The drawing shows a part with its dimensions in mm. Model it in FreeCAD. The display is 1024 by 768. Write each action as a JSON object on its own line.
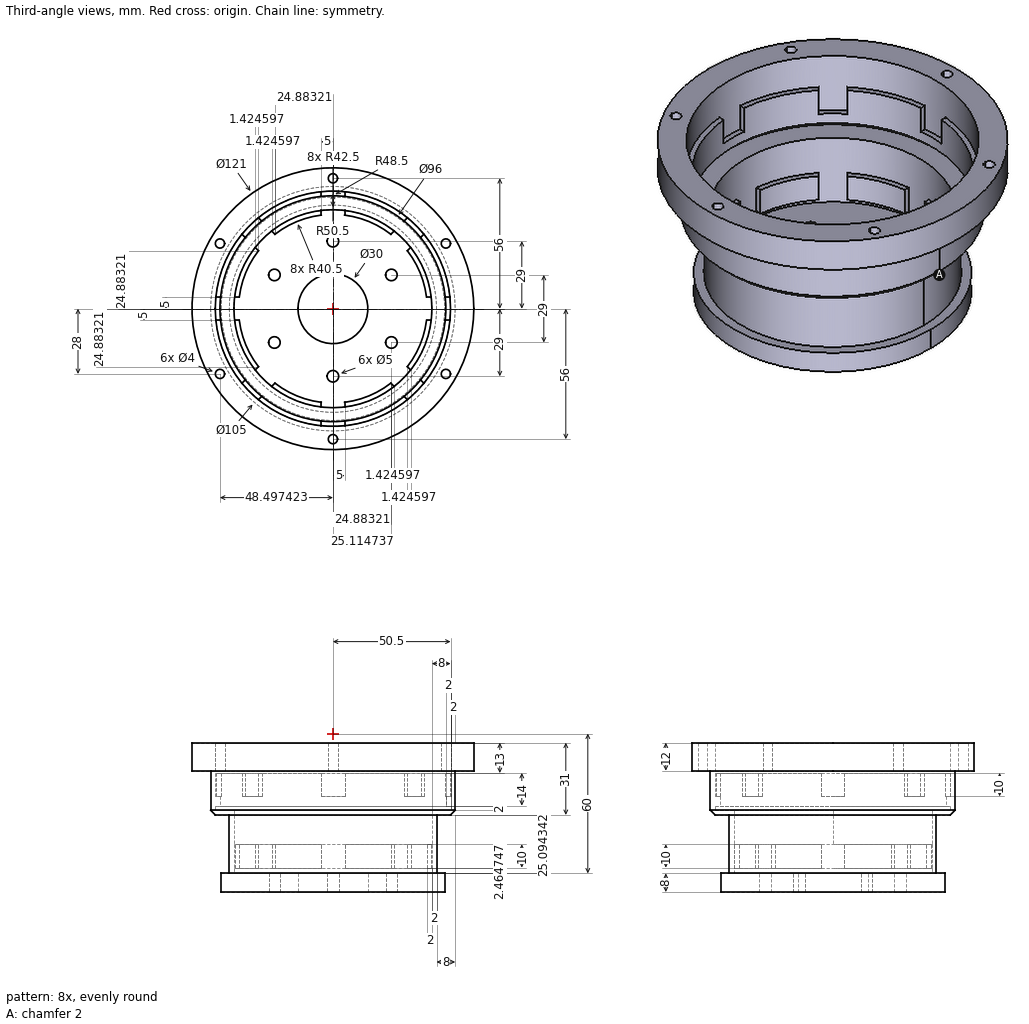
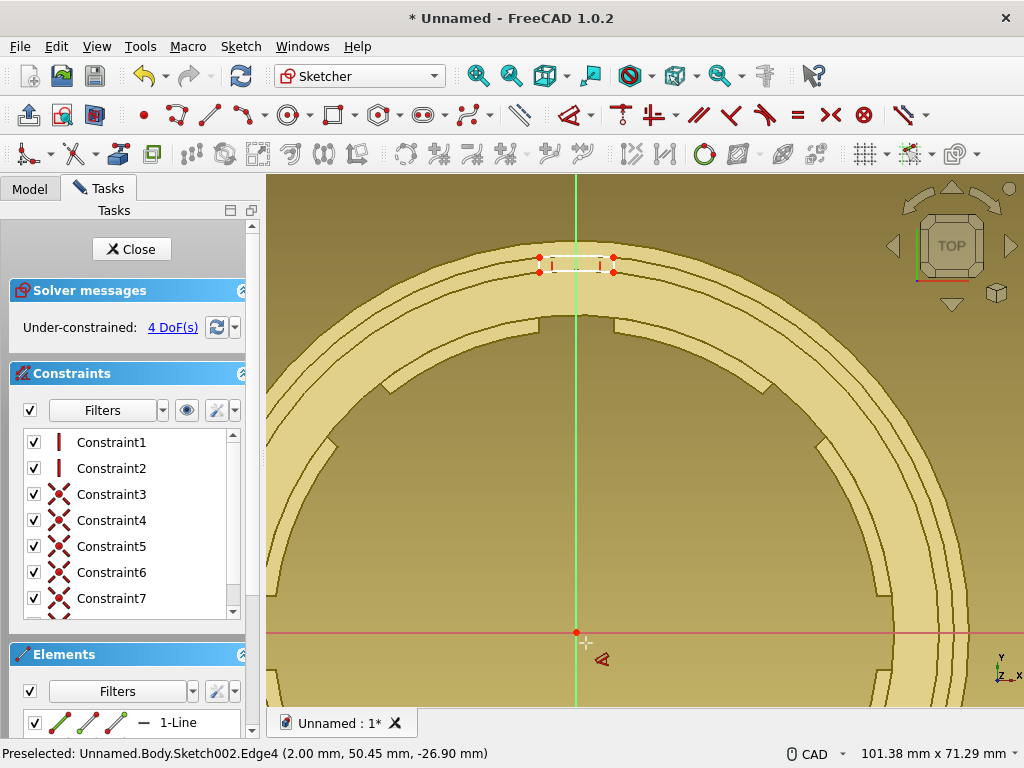
{"action": "left_click", "coordinate": [591, 271]}
{"action": "left_click", "coordinate": [592, 239]}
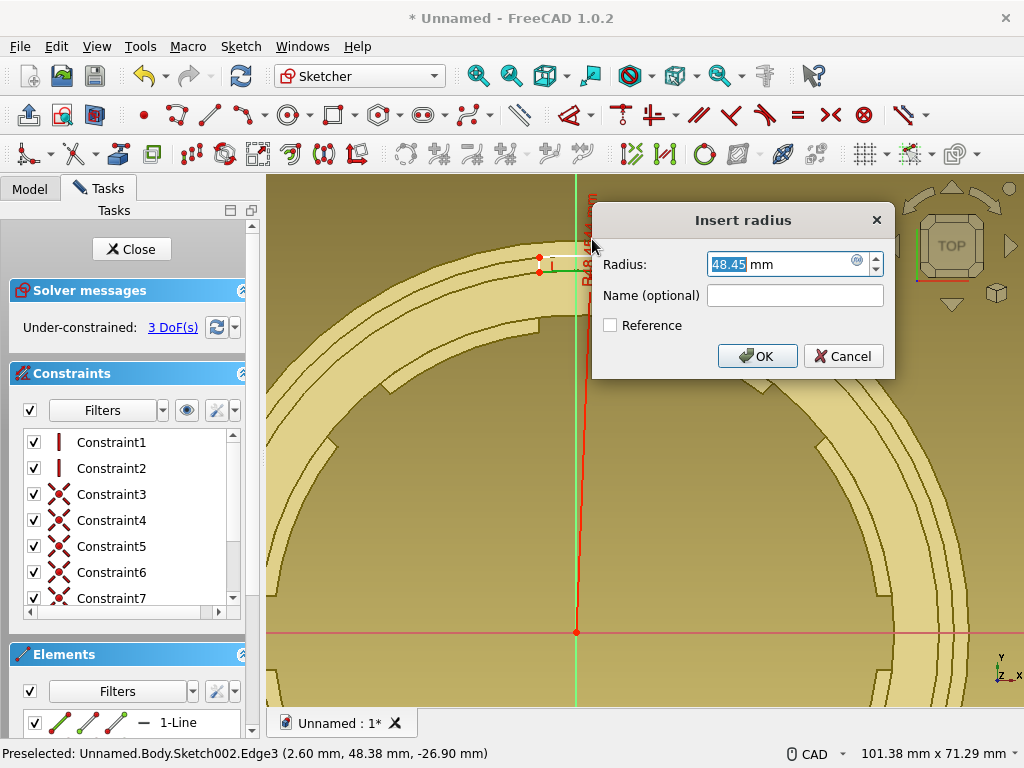
{"action": "type", "text": "48.5"}
{"action": "key", "text": "Return"}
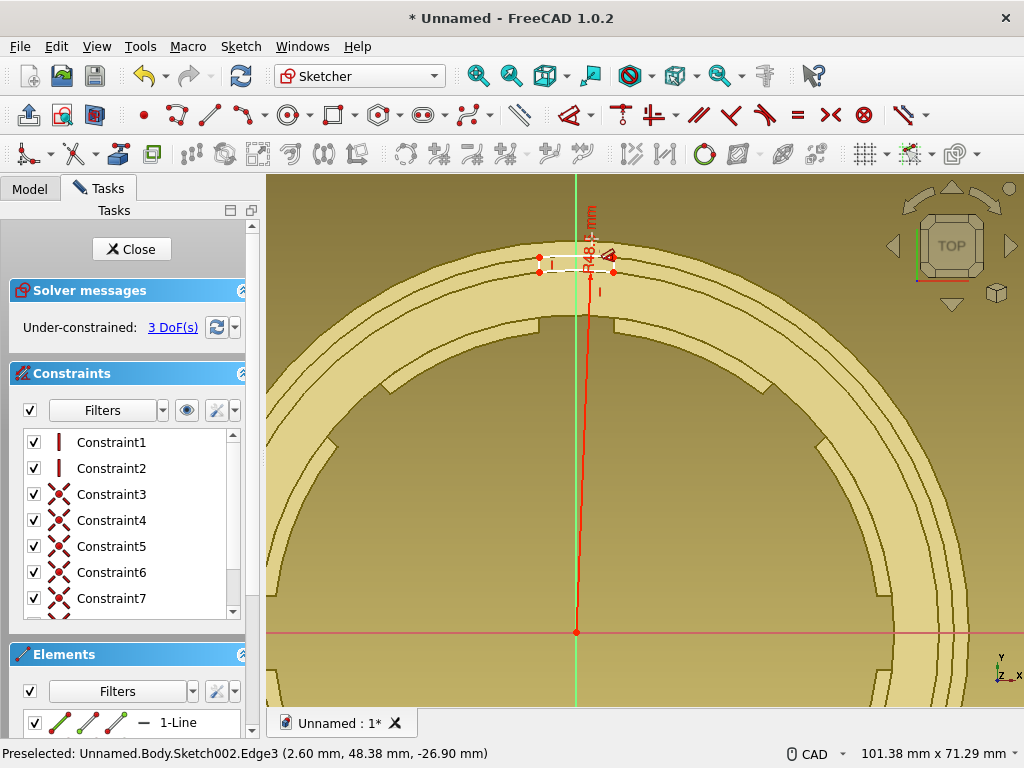
{"action": "left_click", "coordinate": [591, 256]}
{"action": "left_click", "coordinate": [786, 282]}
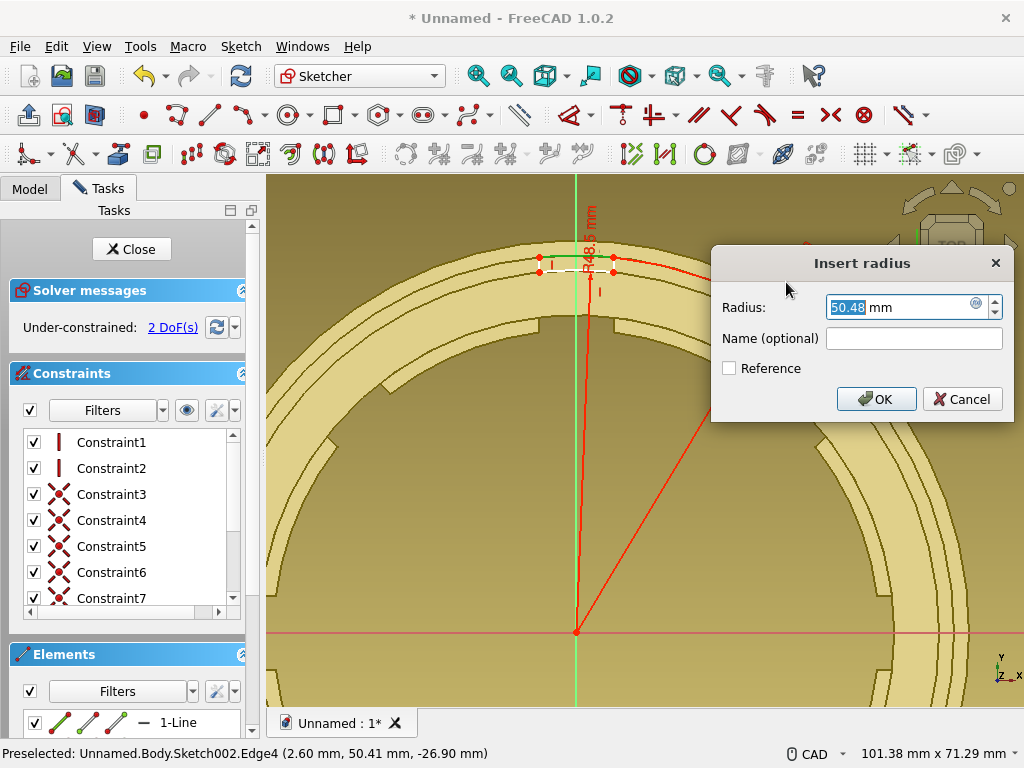
{"action": "type", "text": "50.5"}
{"action": "key", "text": "Return"}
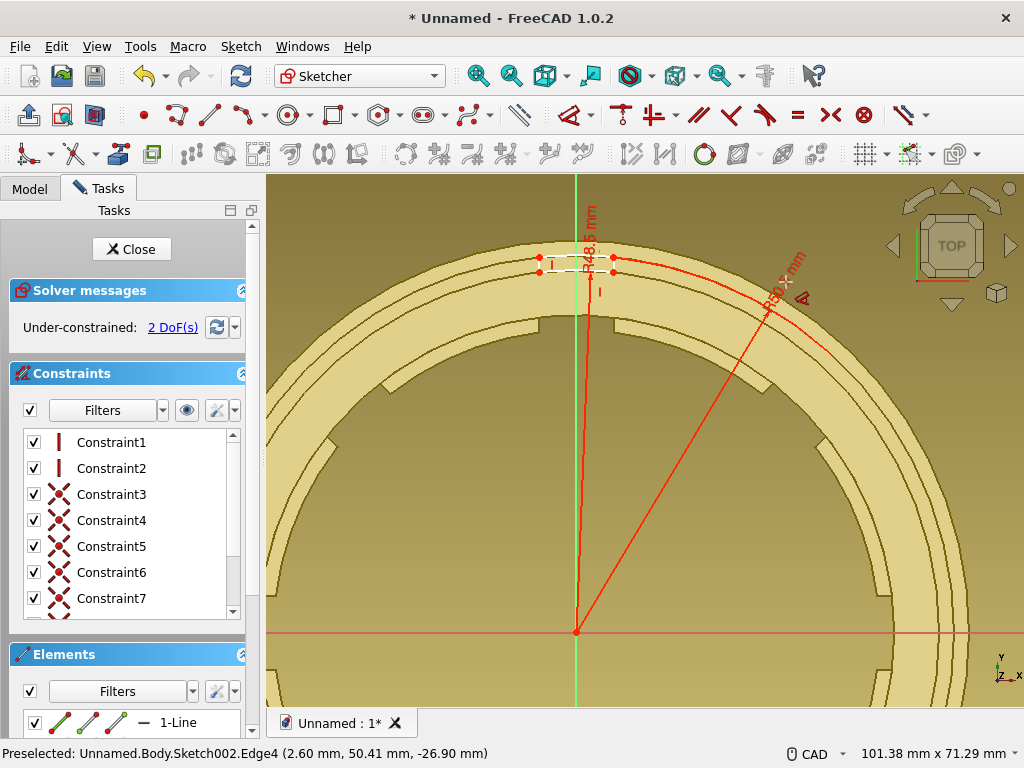
{"action": "left_click", "coordinate": [539, 257]}
{"action": "left_click", "coordinate": [558, 667]}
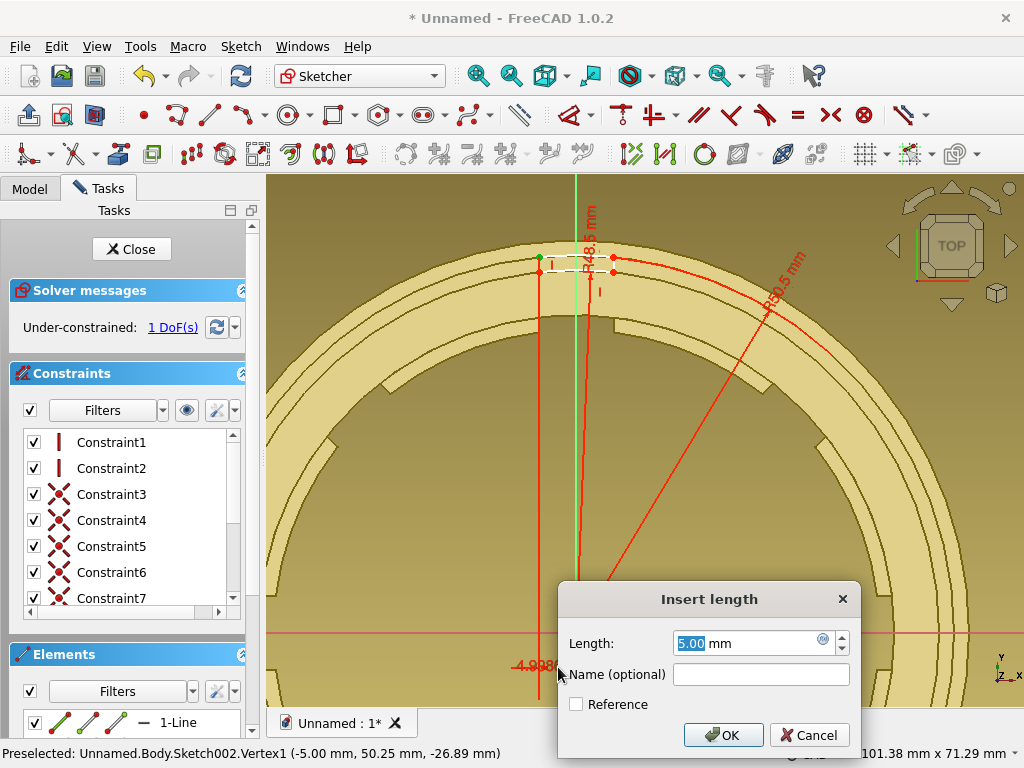
{"action": "type", "text": "5"}
{"action": "key", "text": "Return"}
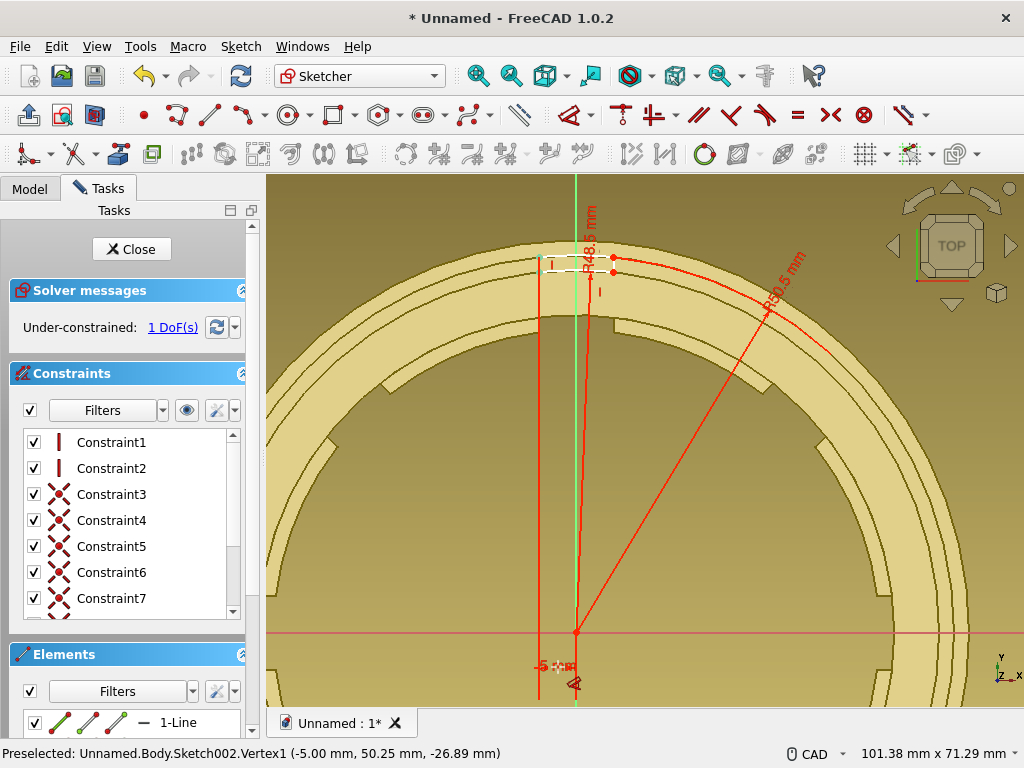
{"action": "left_click", "coordinate": [614, 272]}
{"action": "left_click", "coordinate": [595, 214]}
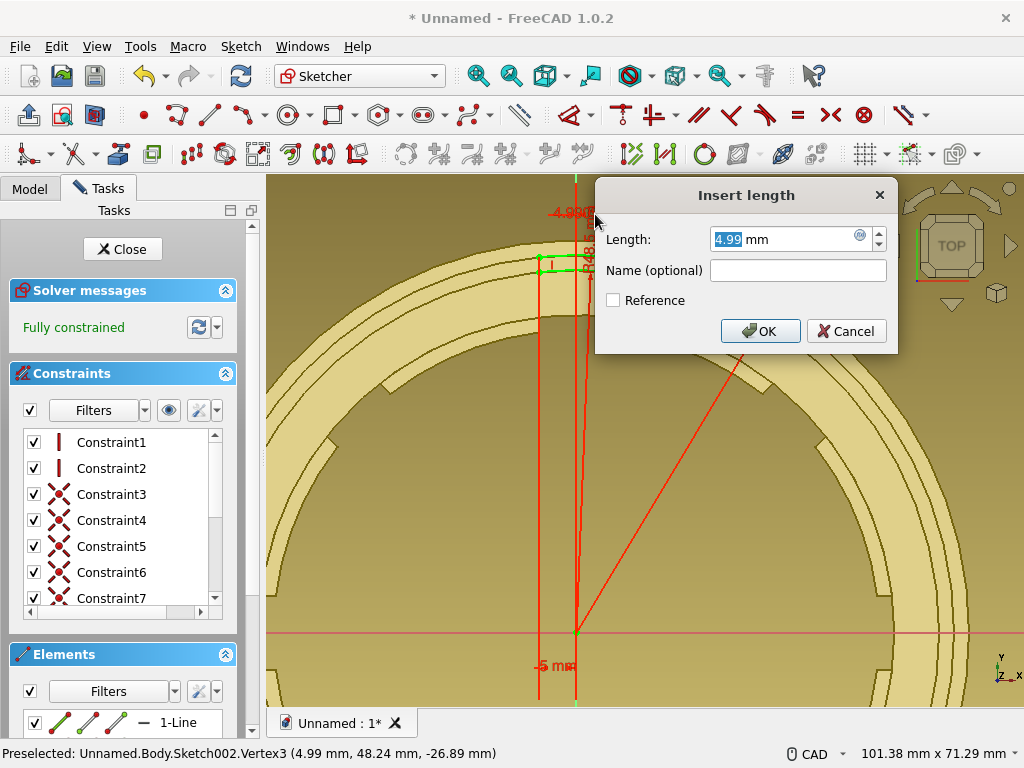
{"action": "type", "text": "5"}
{"action": "key", "text": "Return"}
{"action": "key", "text": "Escape"}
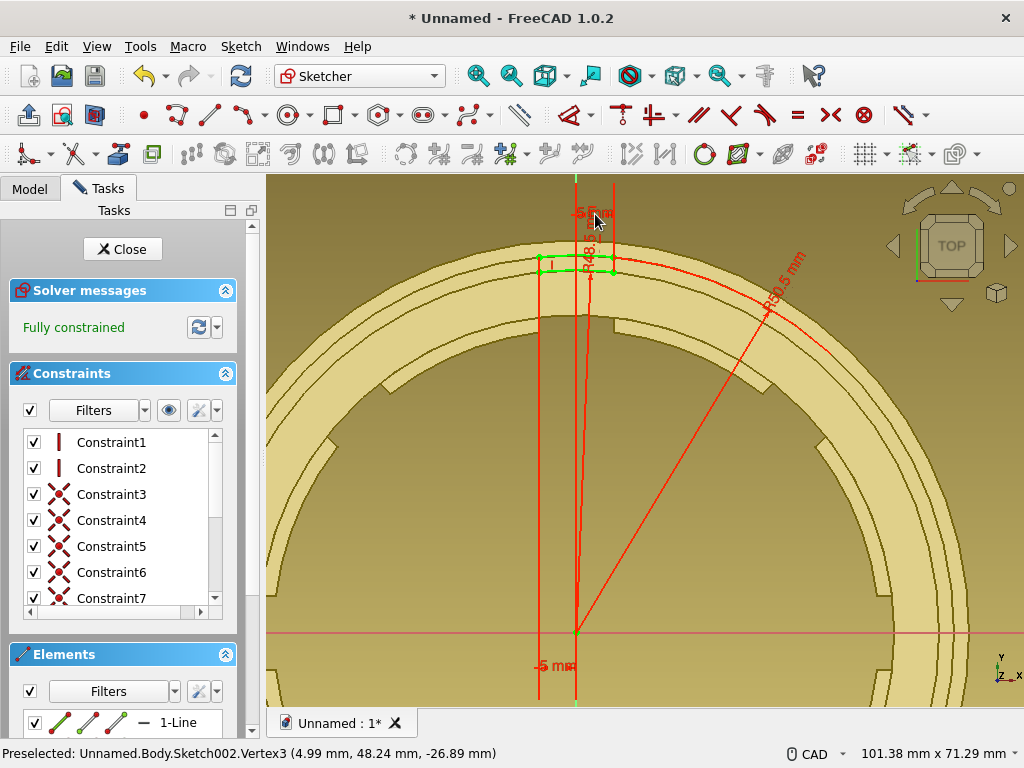
{"action": "left_click", "coordinate": [123, 249]}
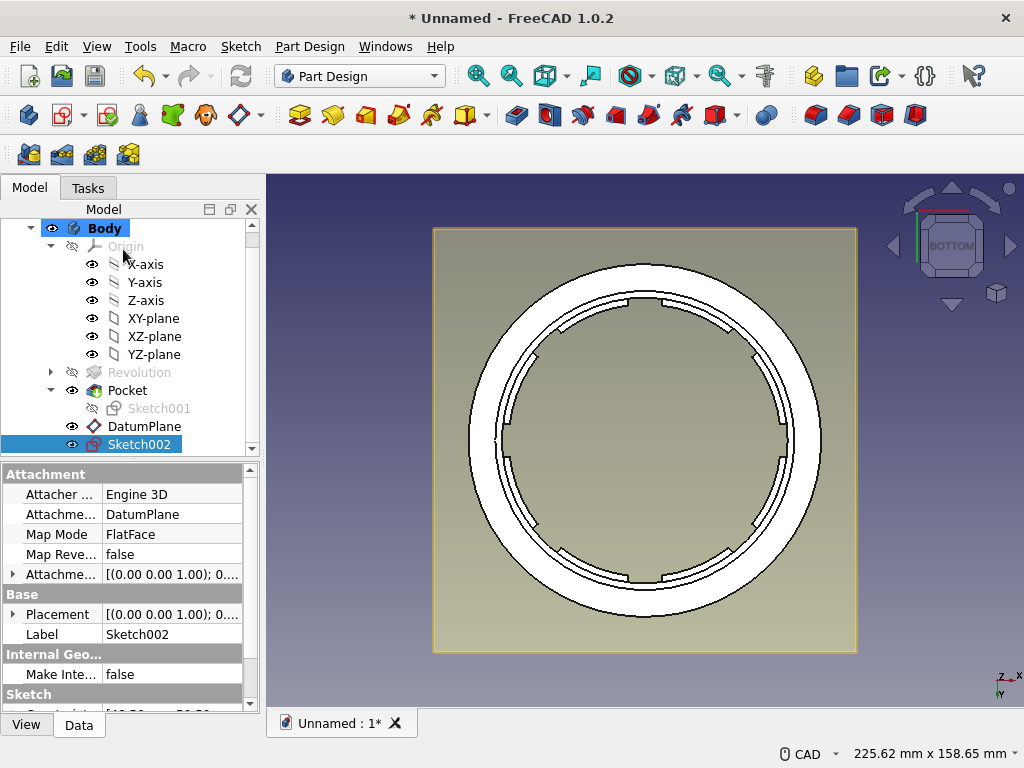
{"action": "left_click", "coordinate": [517, 116]}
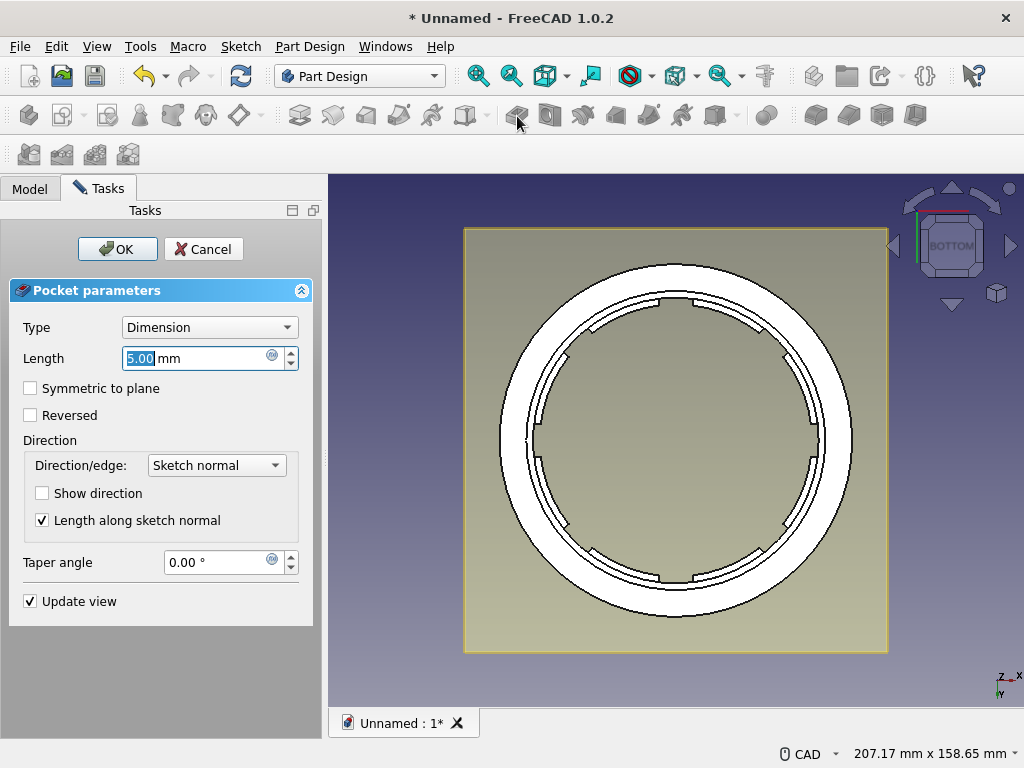
{"action": "type", "text": "10"}
{"action": "key", "text": "Tab"}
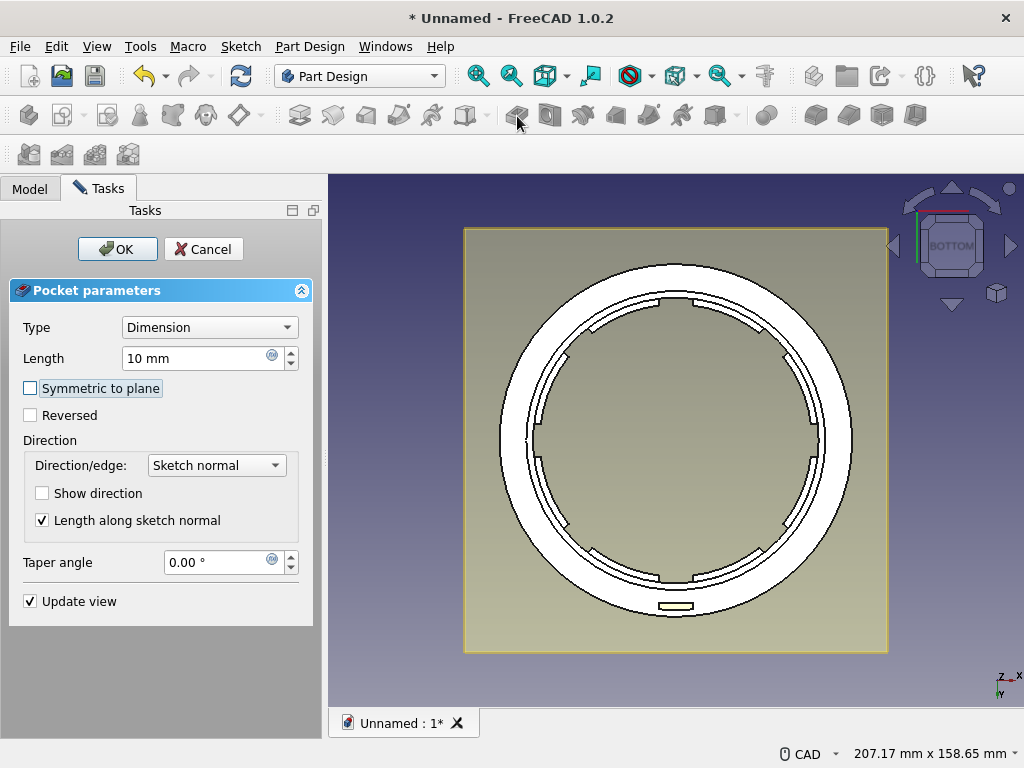
{"action": "left_click", "coordinate": [31, 415]}